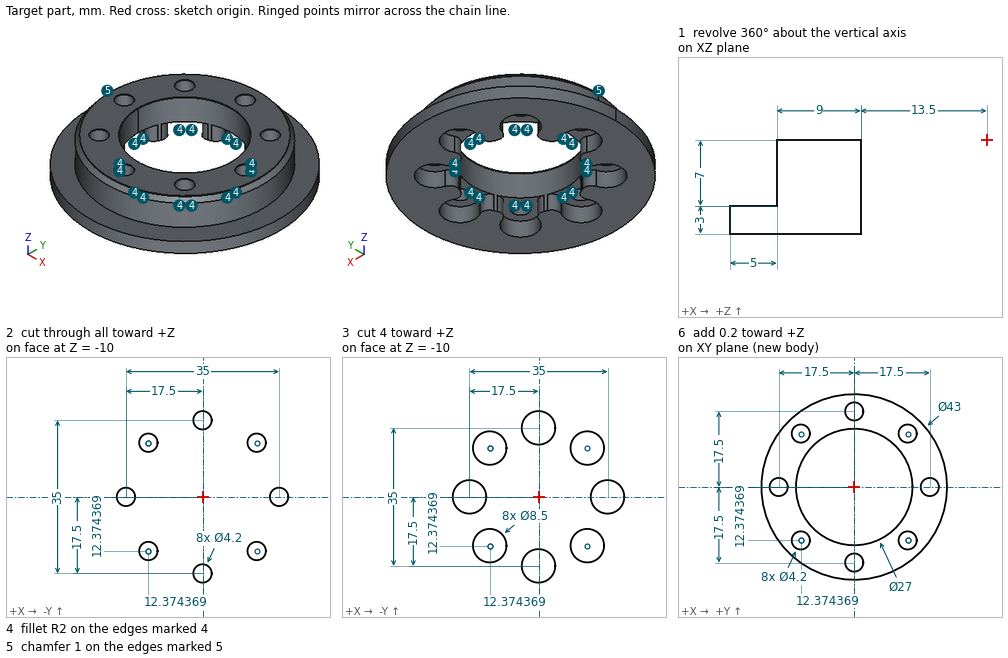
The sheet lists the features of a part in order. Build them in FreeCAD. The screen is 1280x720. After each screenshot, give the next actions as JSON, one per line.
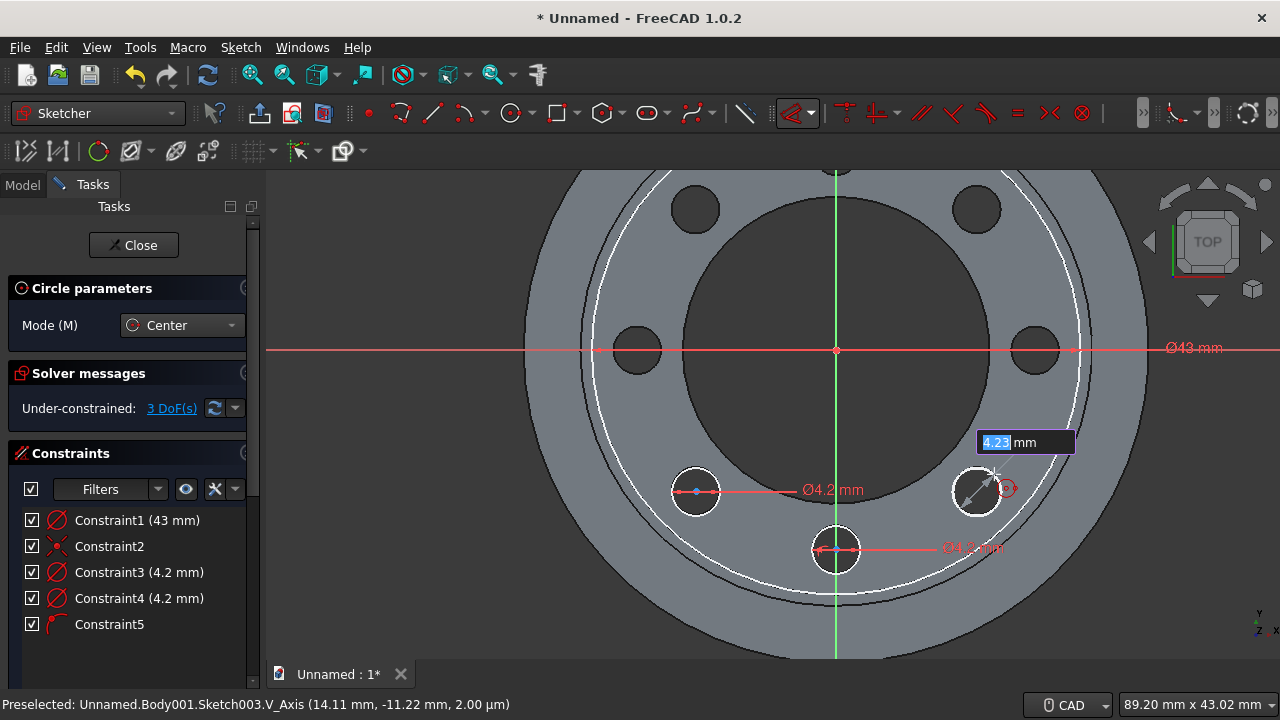
{"action": "type", "text": "4.2"}
{"action": "key", "text": "Return"}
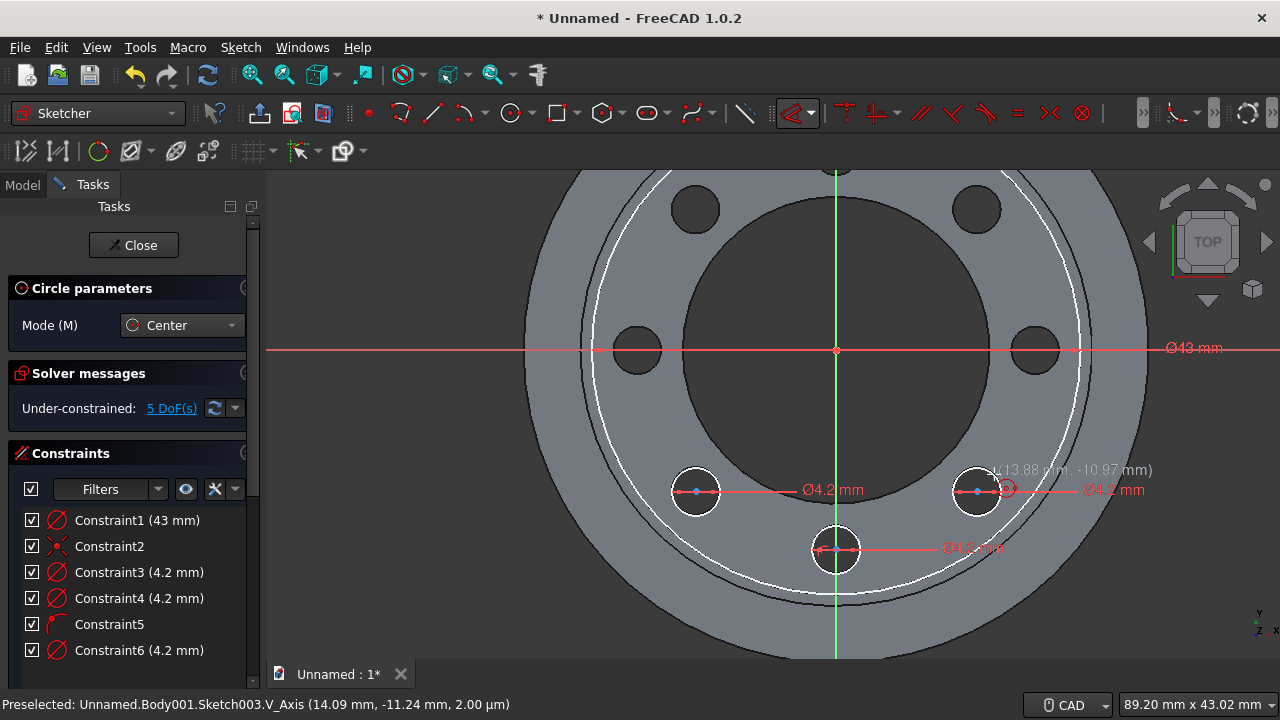
{"action": "left_click", "coordinate": [637, 350]}
{"action": "mouse_move", "coordinate": [654, 333]}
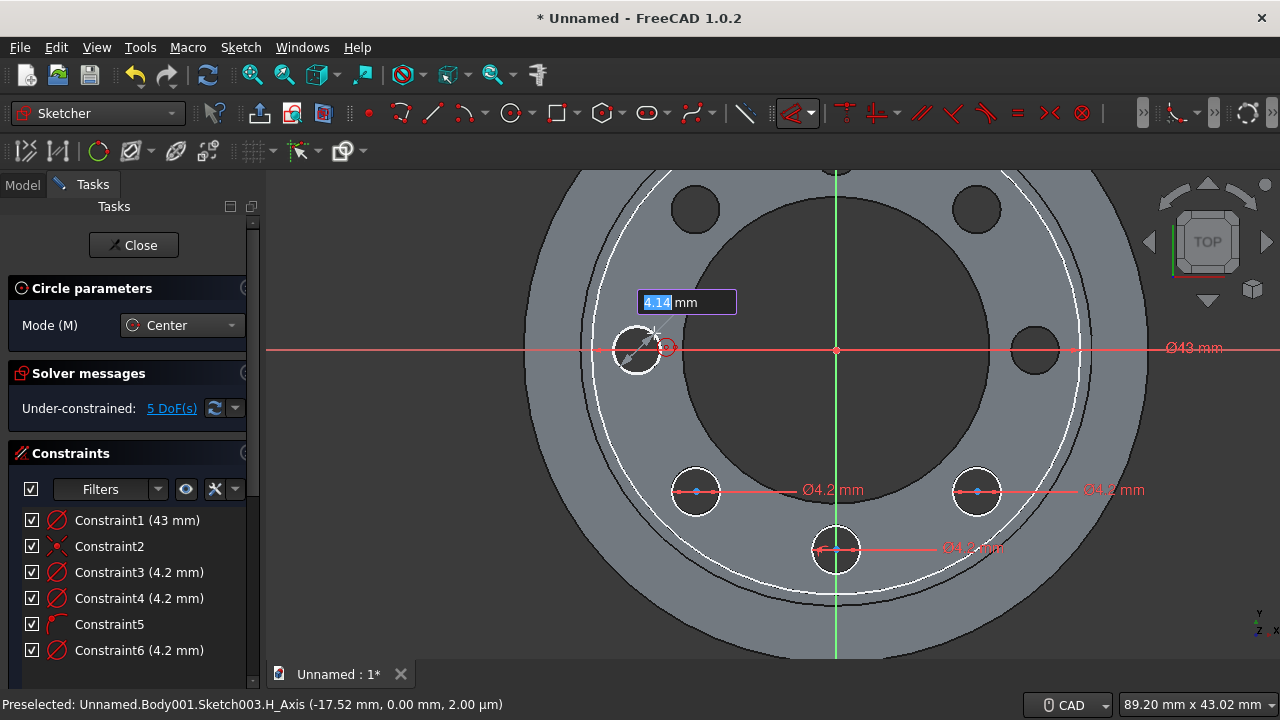
{"action": "type", "text": "4.2"}
{"action": "key", "text": "Return"}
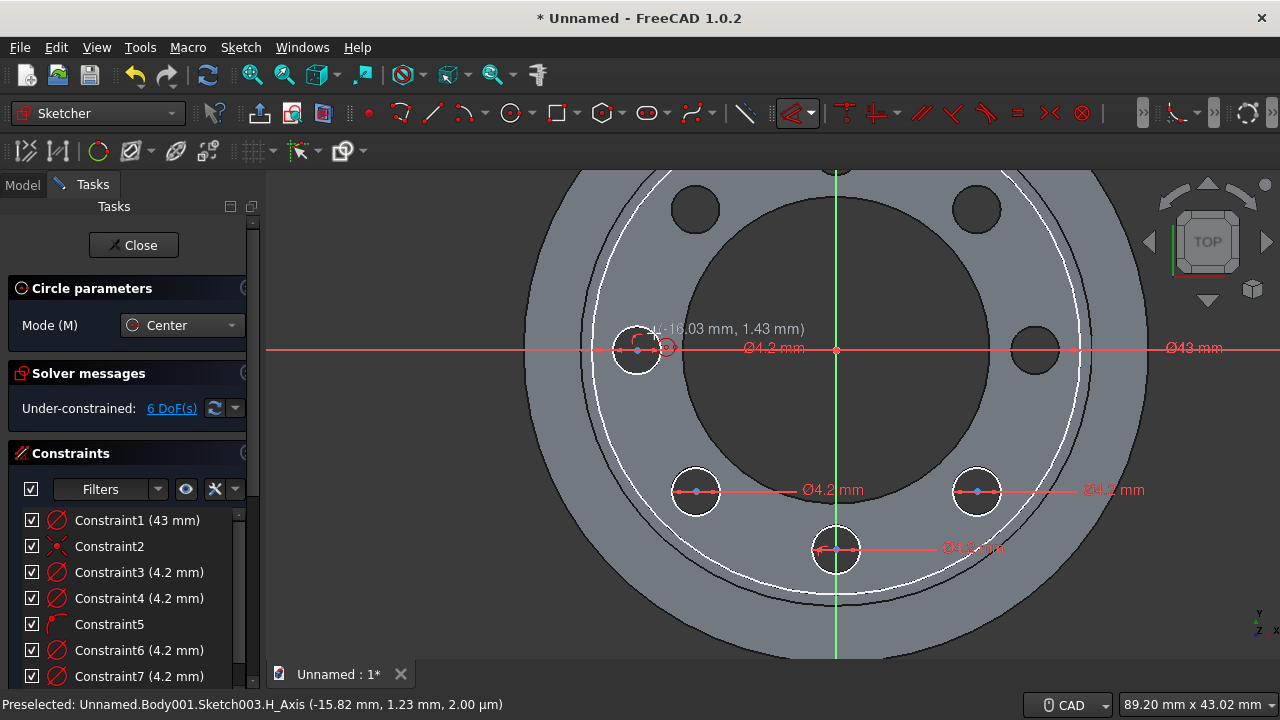
{"action": "left_click", "coordinate": [696, 210]}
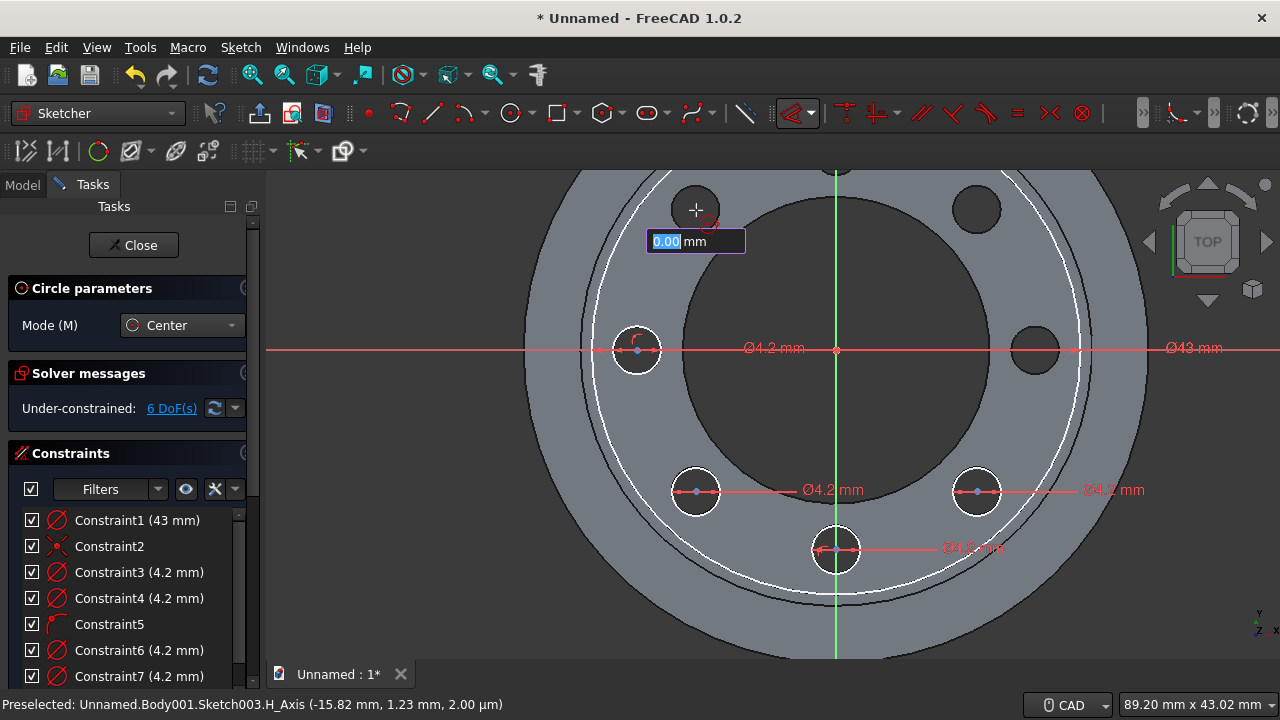
{"action": "scroll", "coordinate": [437, 545], "scroll_direction": "down", "scroll_amount": 2}
{"action": "mouse_move", "coordinate": [622, 309]}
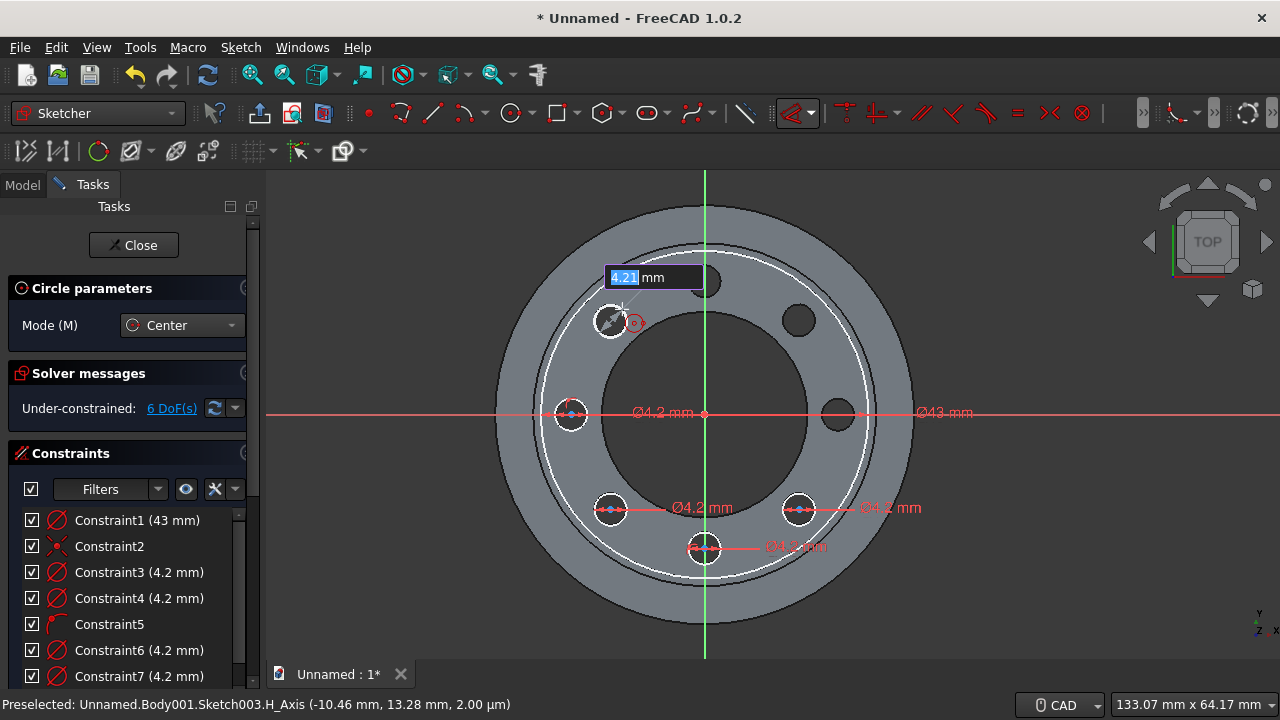
{"action": "type", "text": "4.2"}
{"action": "key", "text": "Return"}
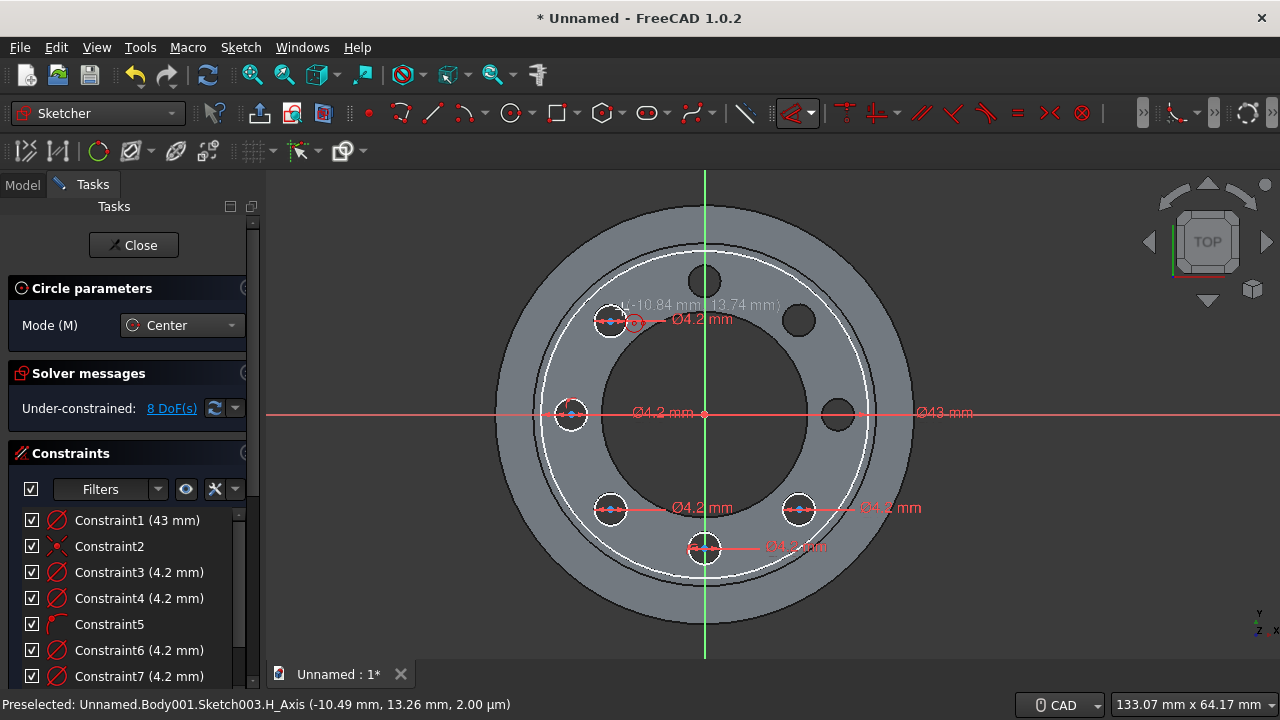
{"action": "left_click", "coordinate": [705, 415]}
{"action": "mouse_move", "coordinate": [777, 342]}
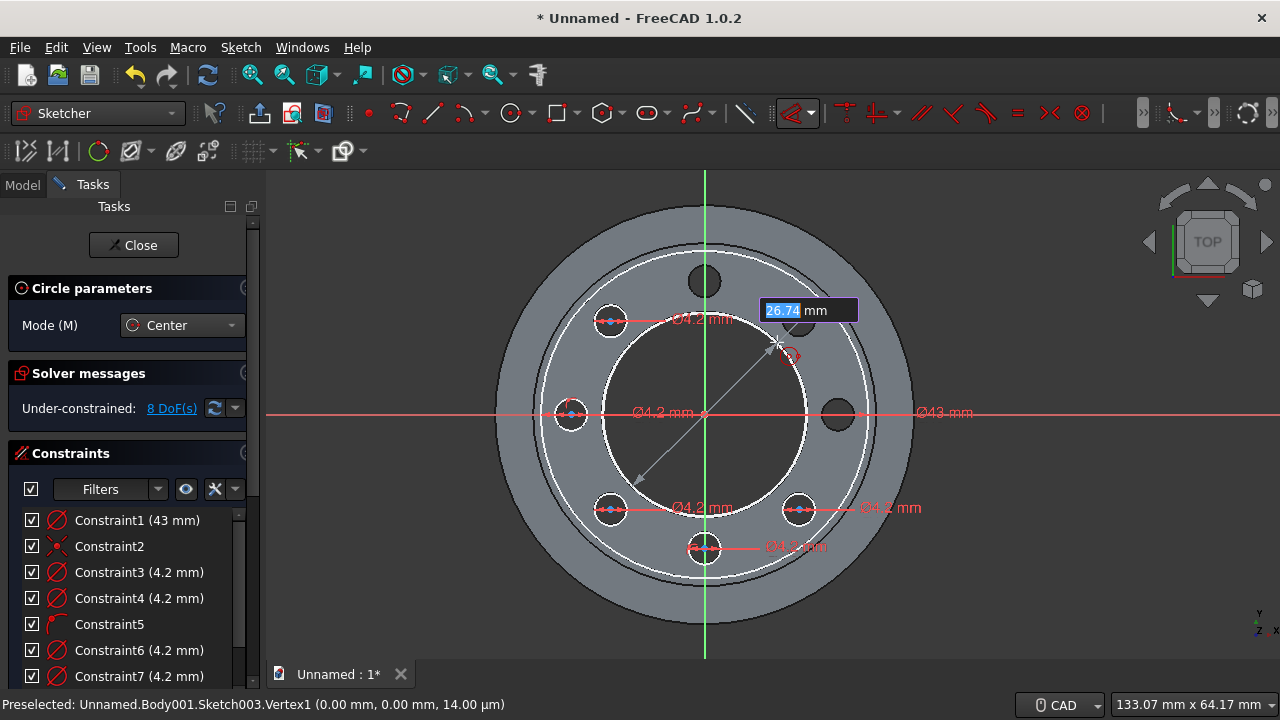
{"action": "type", "text": "27"}
{"action": "key", "text": "Return"}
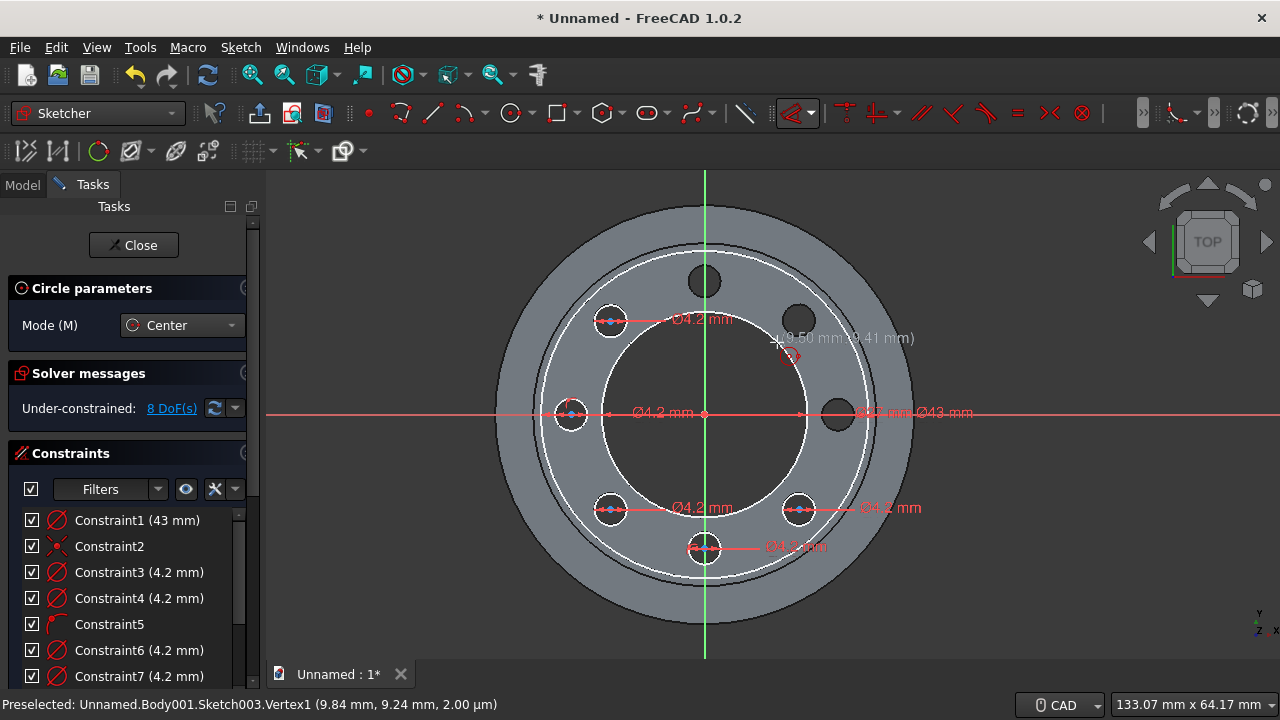
{"action": "scroll", "coordinate": [838, 415], "scroll_direction": "up", "scroll_amount": 2}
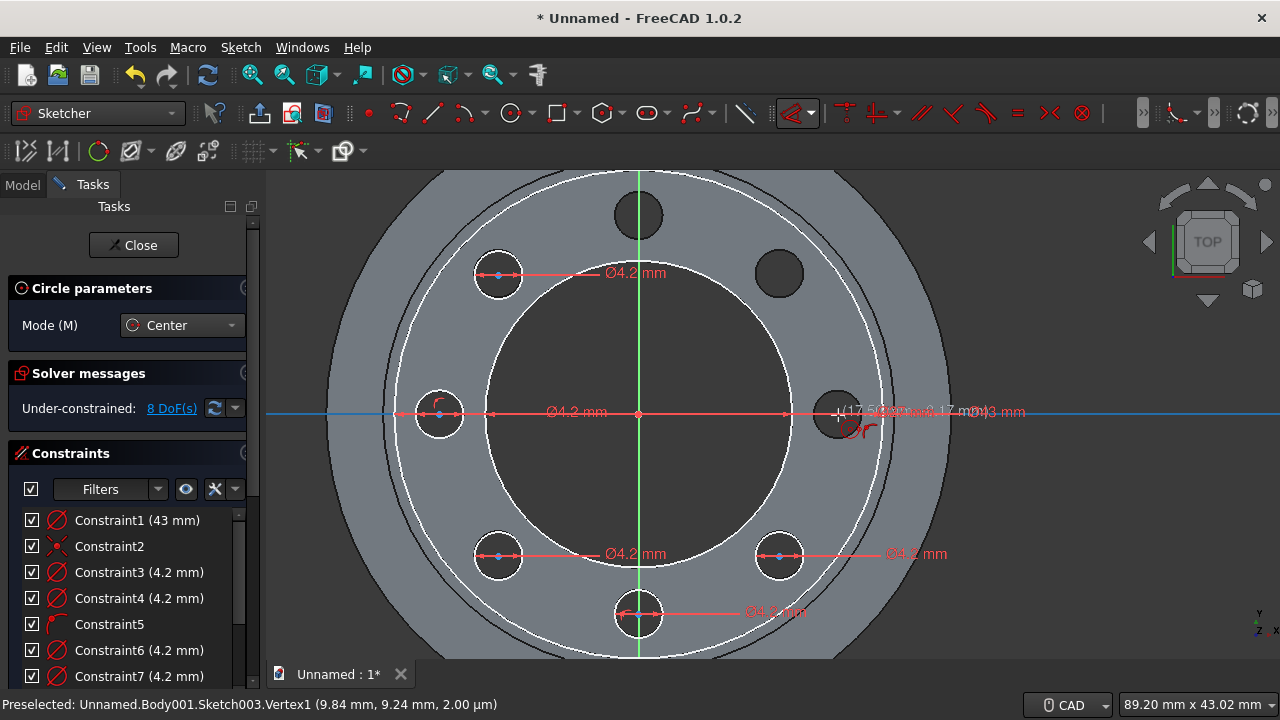
{"action": "left_click", "coordinate": [838, 414]}
{"action": "mouse_move", "coordinate": [855, 397]}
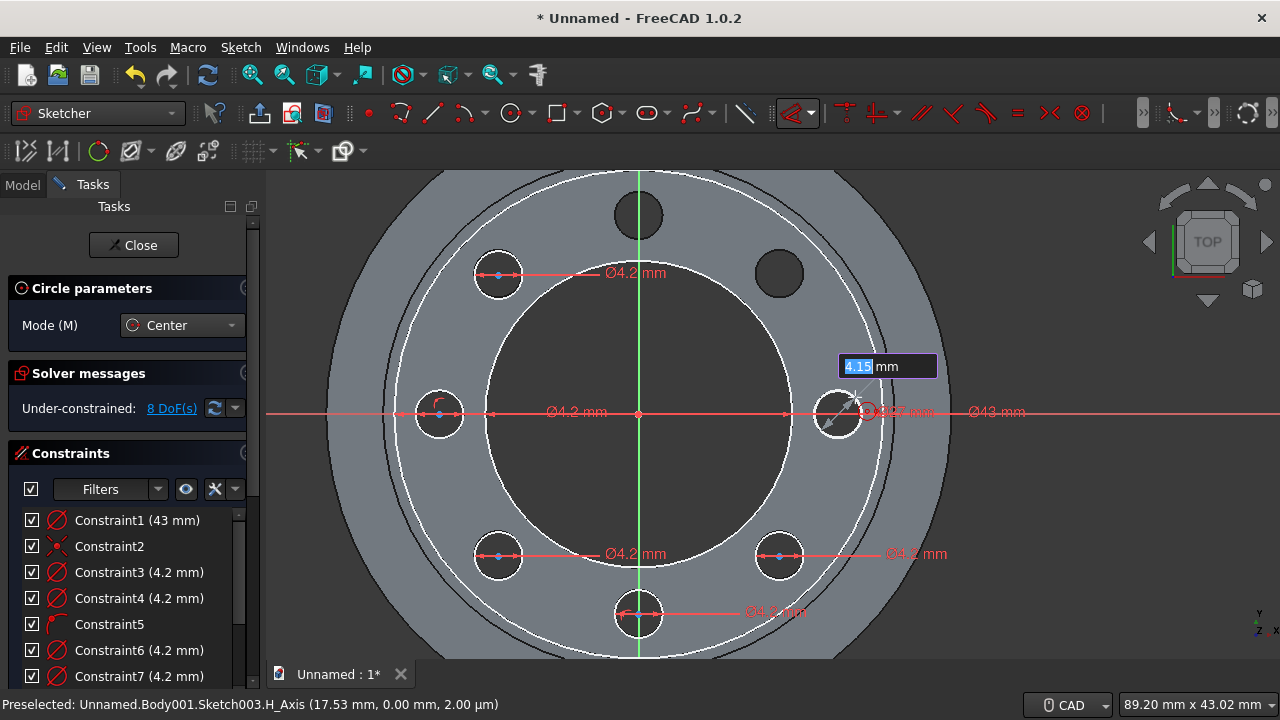
{"action": "type", "text": "4.2"}
{"action": "key", "text": "Return"}